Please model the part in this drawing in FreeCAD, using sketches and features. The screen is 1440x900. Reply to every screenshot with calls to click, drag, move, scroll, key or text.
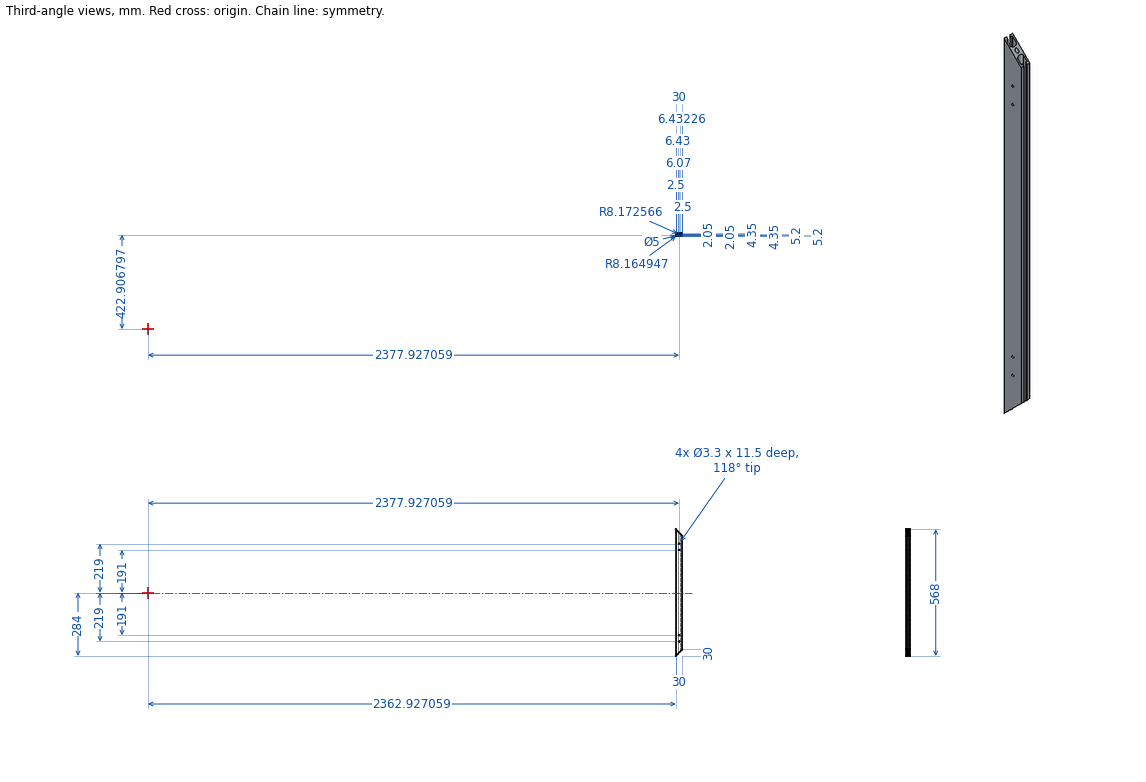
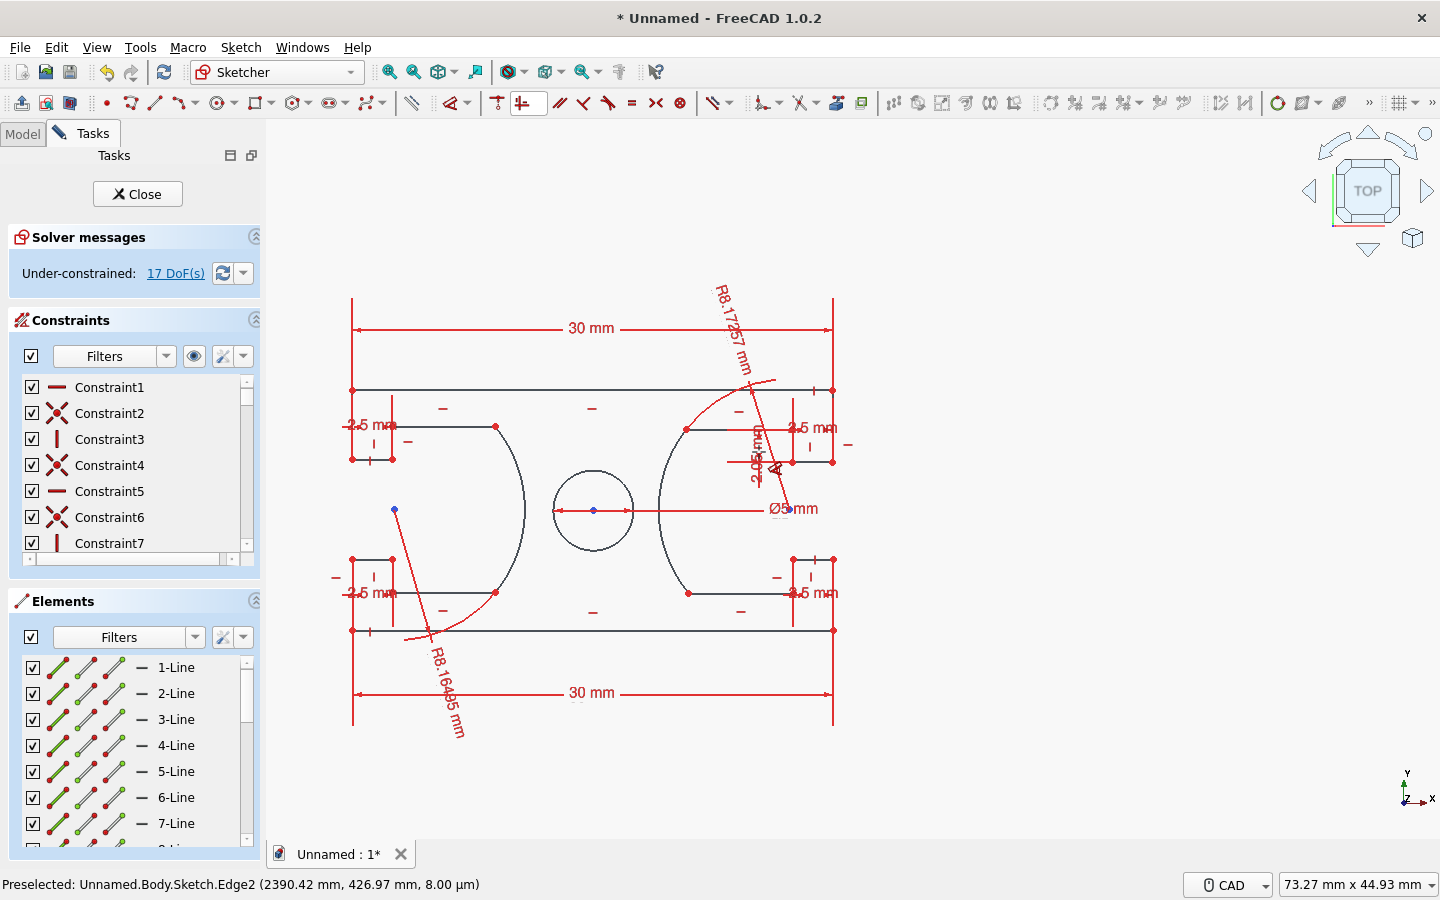
click(833, 441)
click(867, 401)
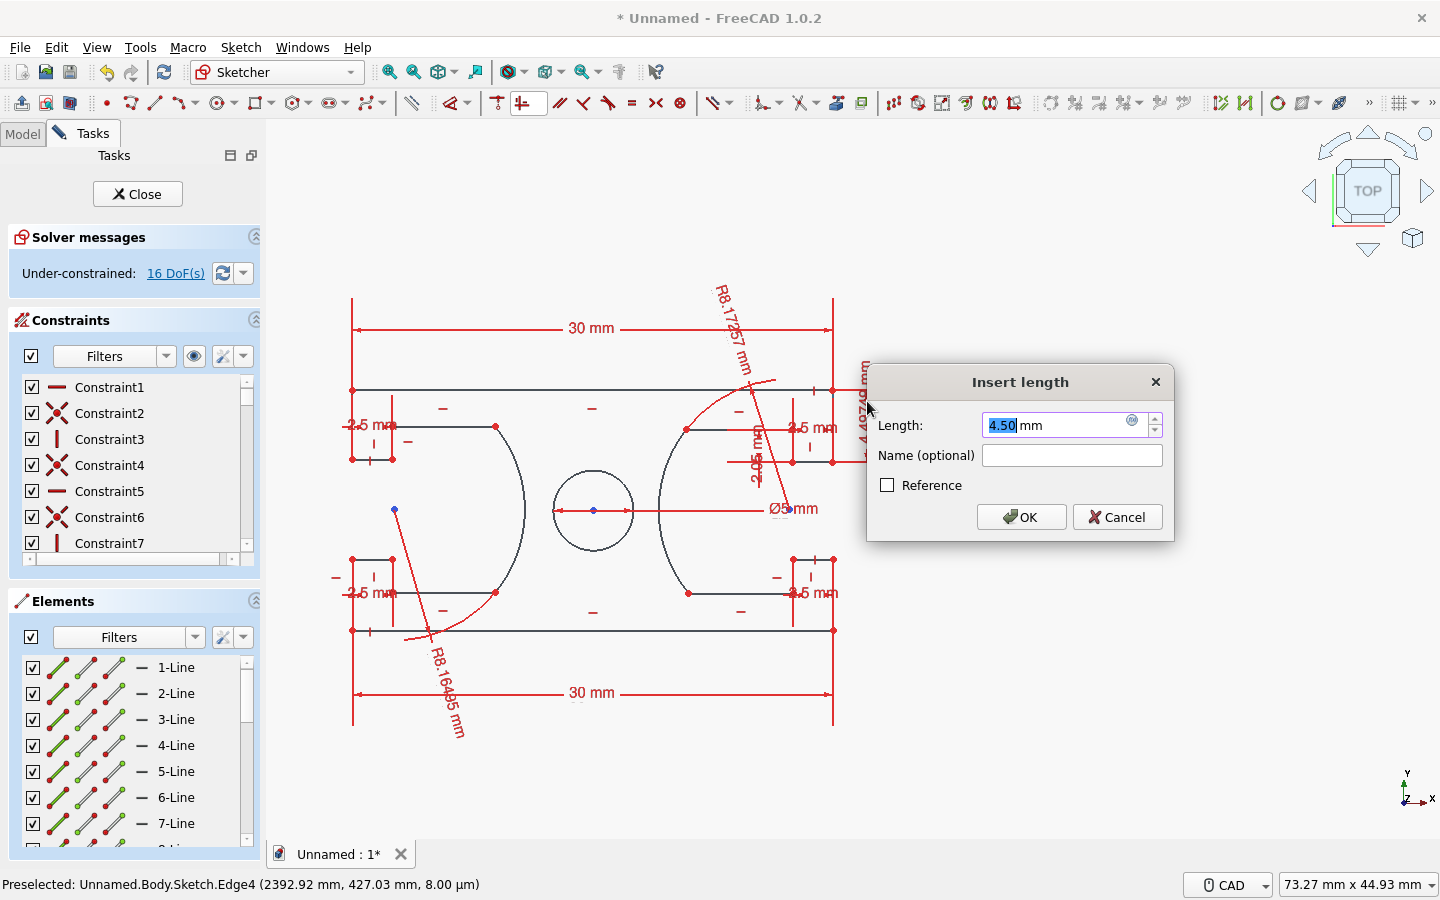
text(4.35)
key(Return)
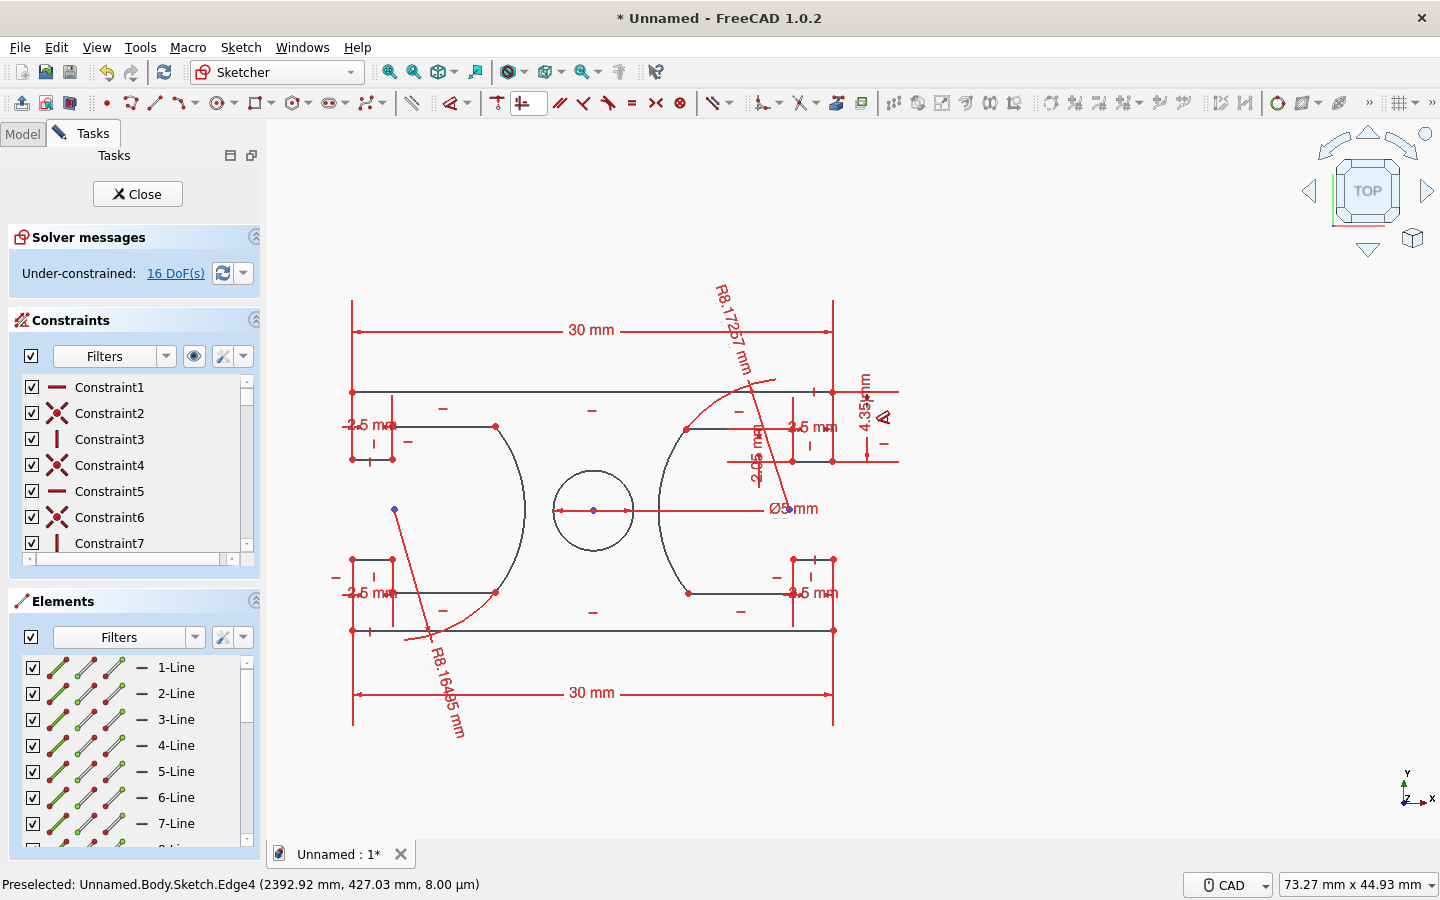
click(352, 412)
click(318, 402)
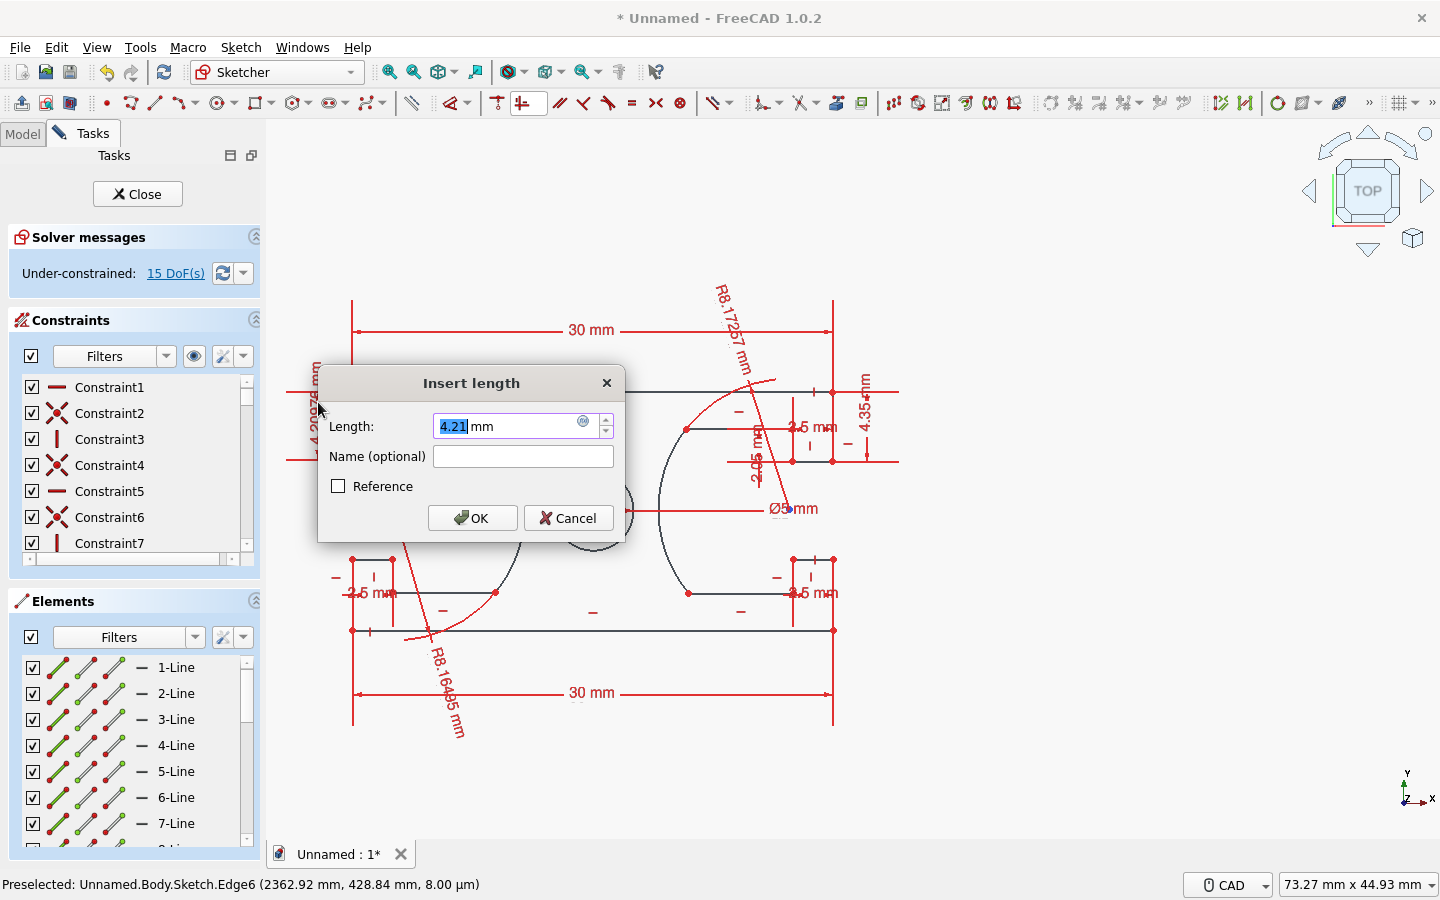
text(4.35)
key(Return)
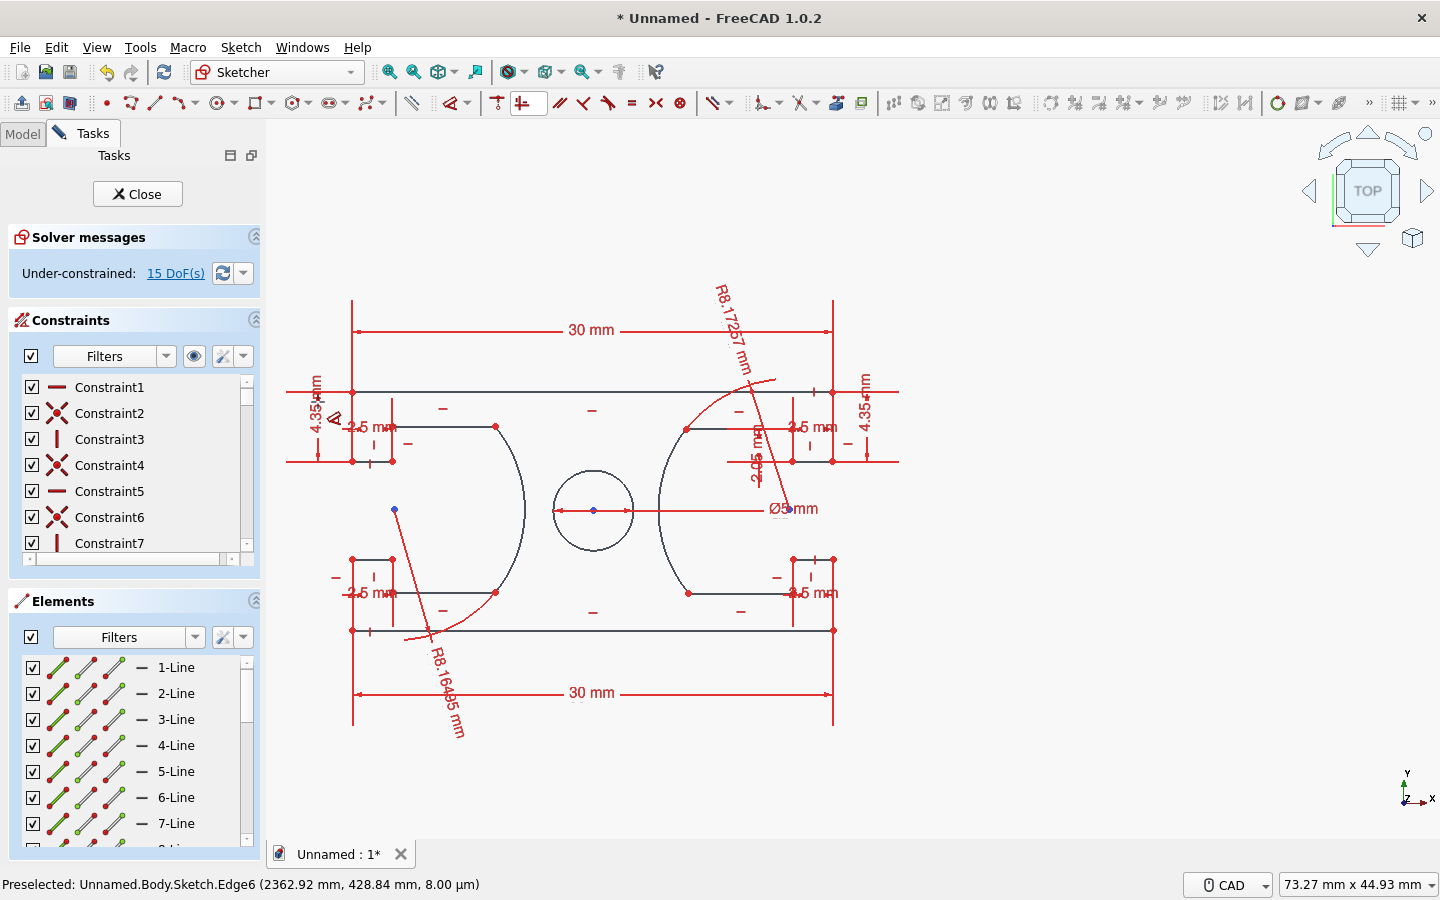
scroll(392, 451, up, 2)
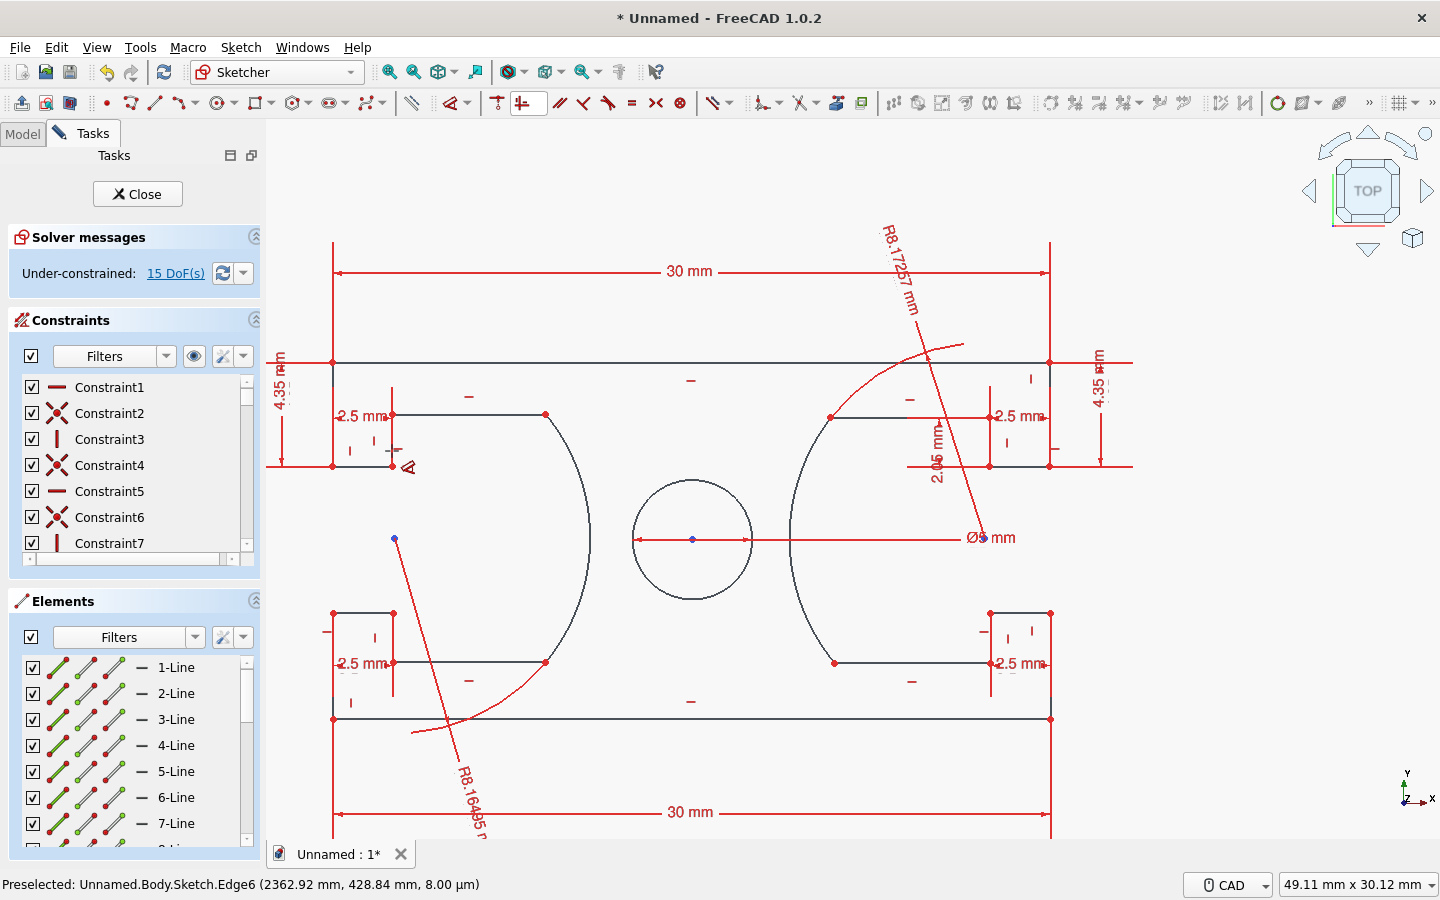
click(392, 451)
click(358, 441)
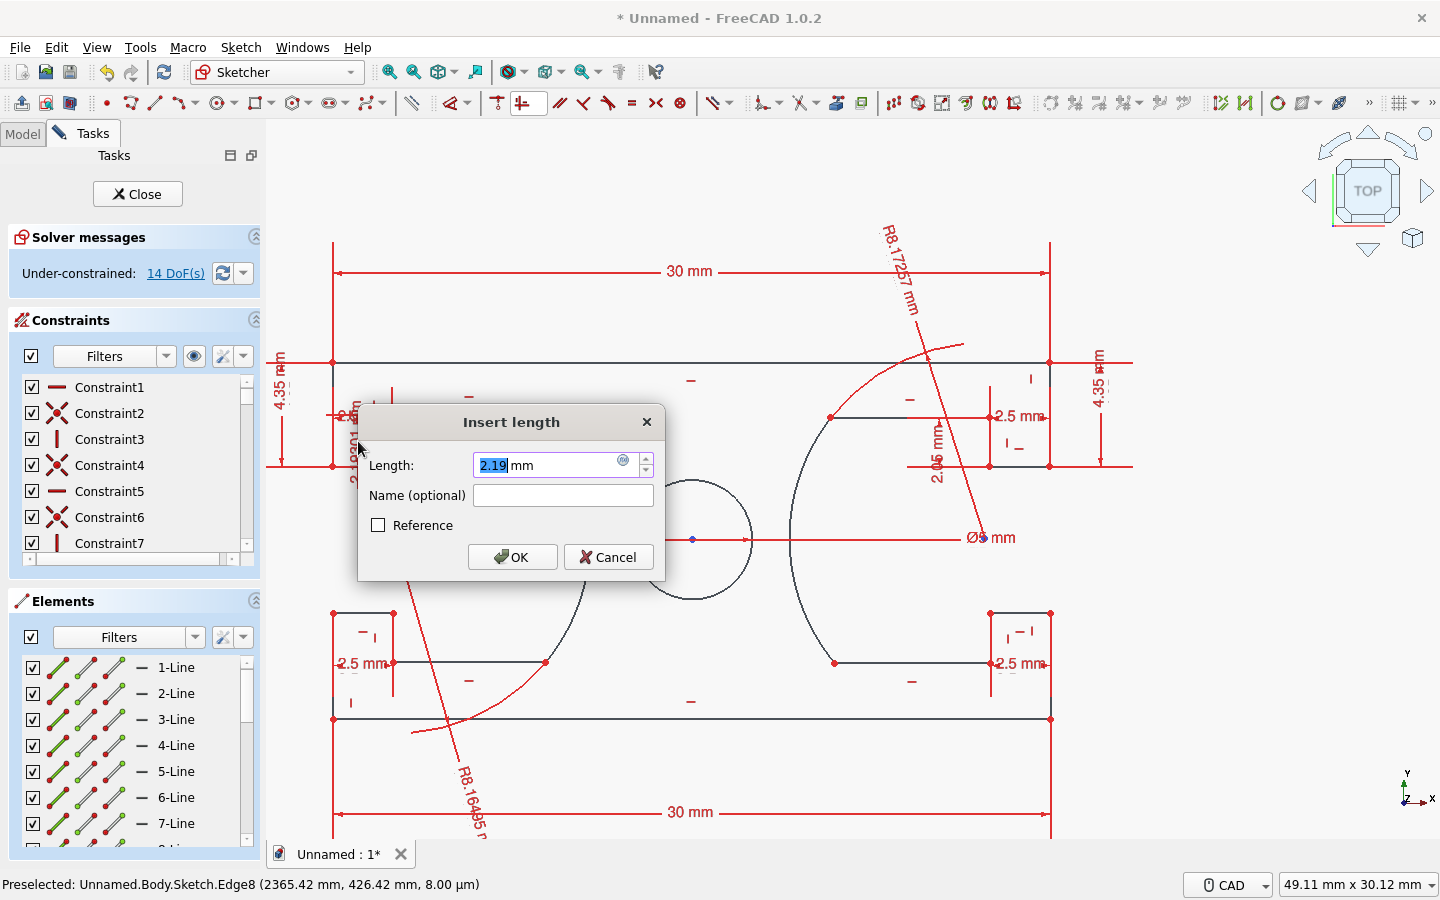
text(2.05)
key(Return)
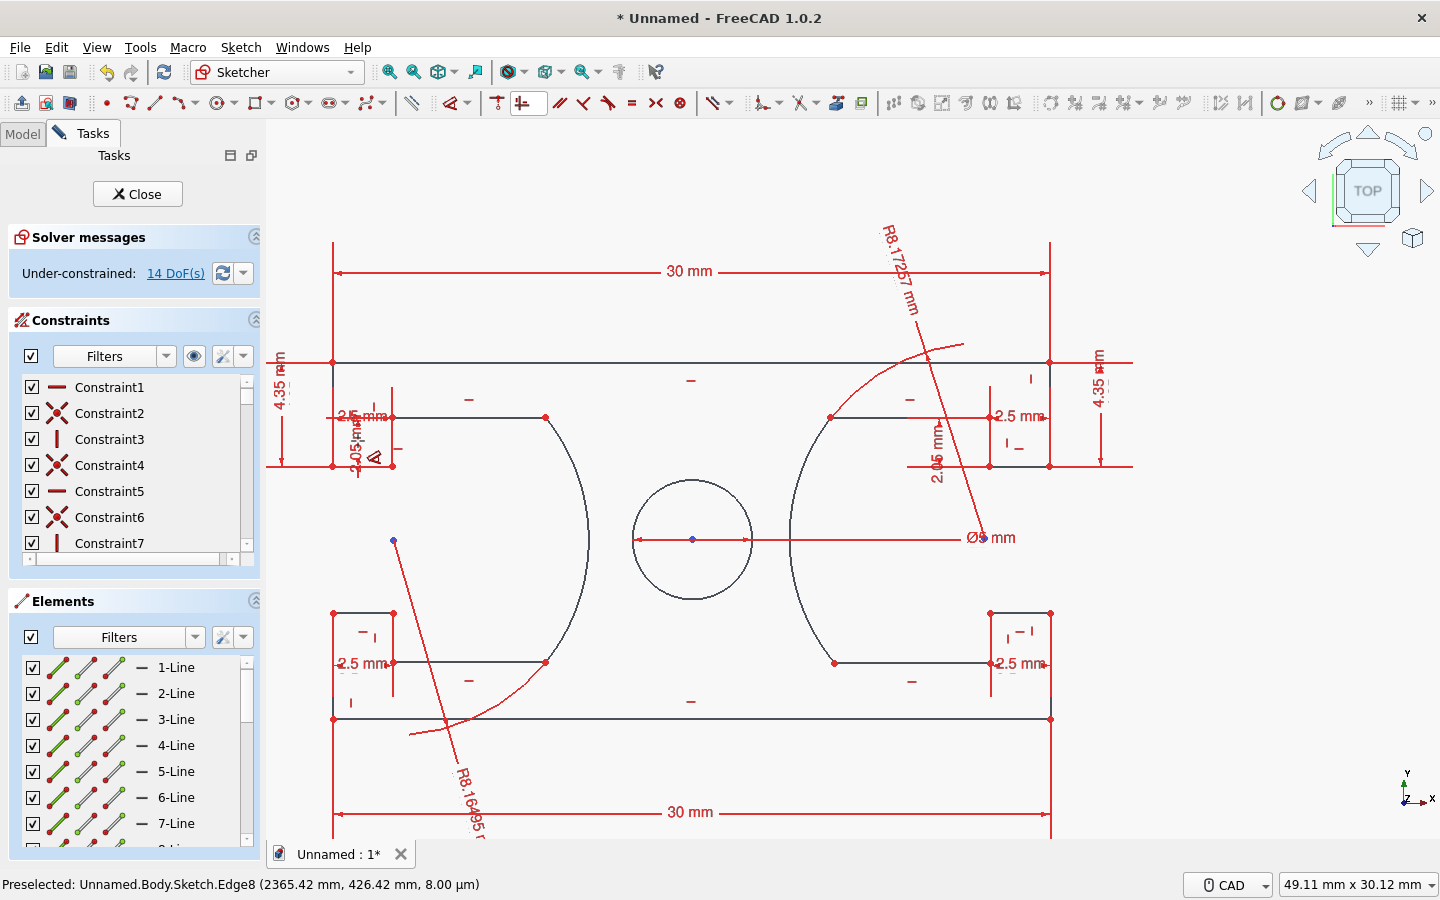
click(438, 418)
click(469, 384)